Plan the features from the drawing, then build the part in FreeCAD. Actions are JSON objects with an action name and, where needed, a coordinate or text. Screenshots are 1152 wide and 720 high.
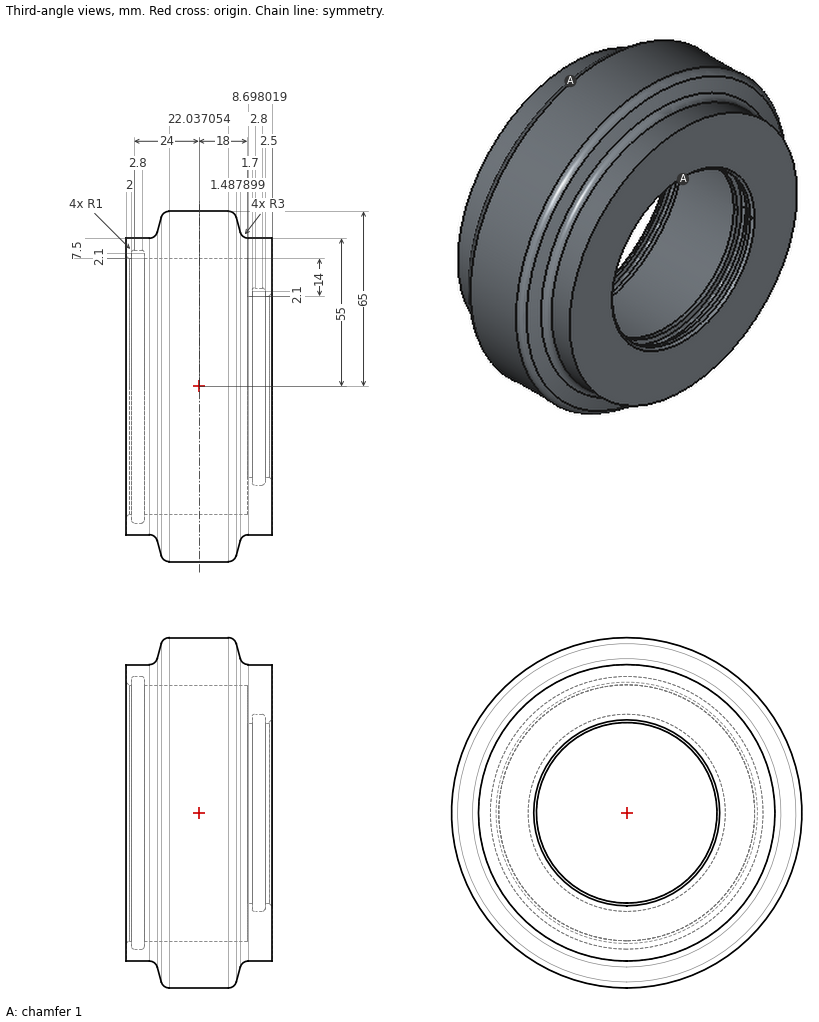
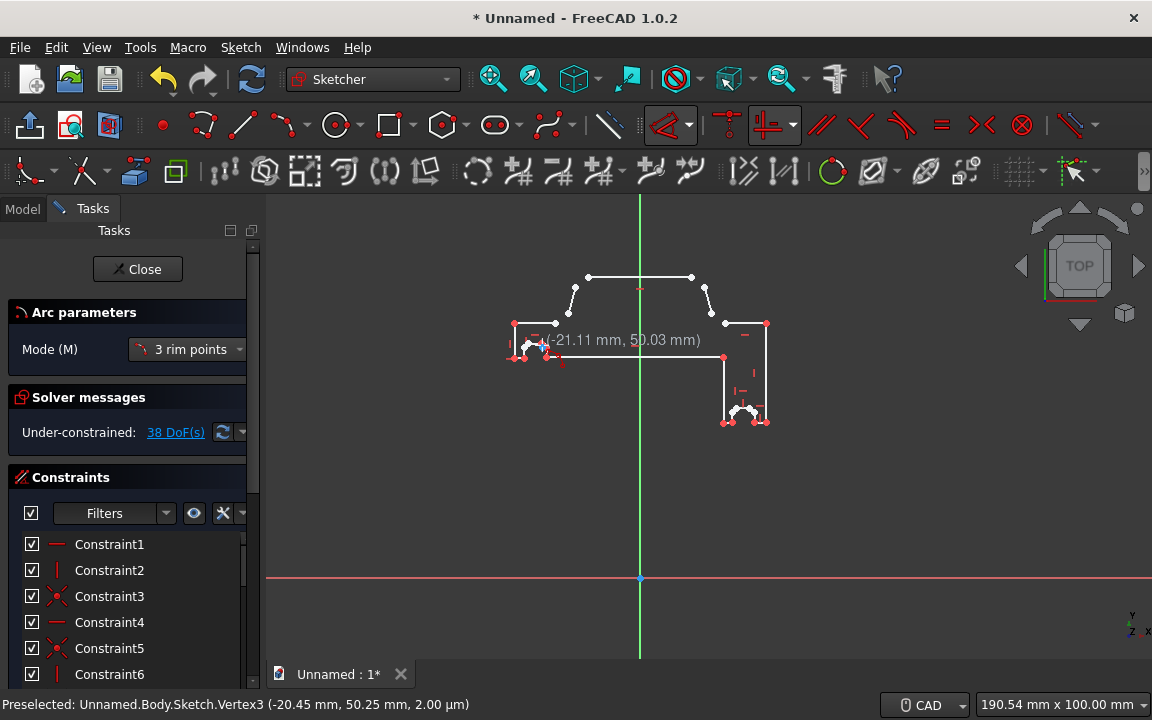
{"action": "scroll", "coordinate": [732, 412], "scroll_direction": "up", "scroll_amount": 6}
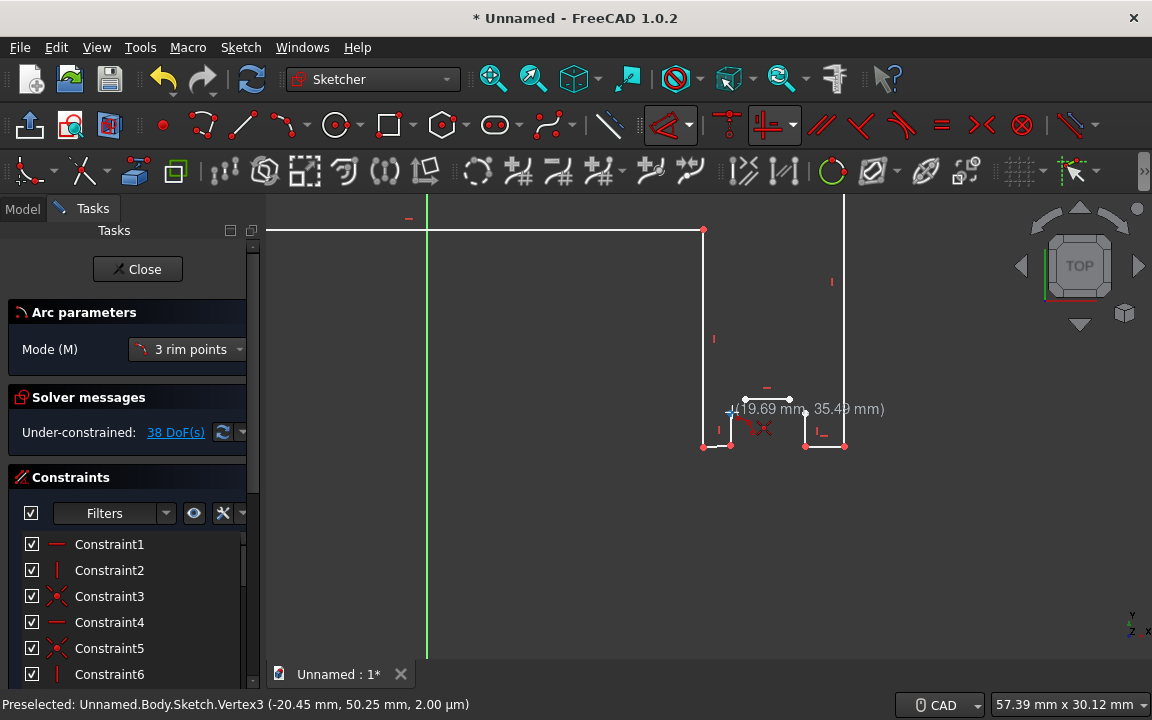
{"action": "left_click", "coordinate": [731, 414]}
{"action": "left_click", "coordinate": [746, 399]}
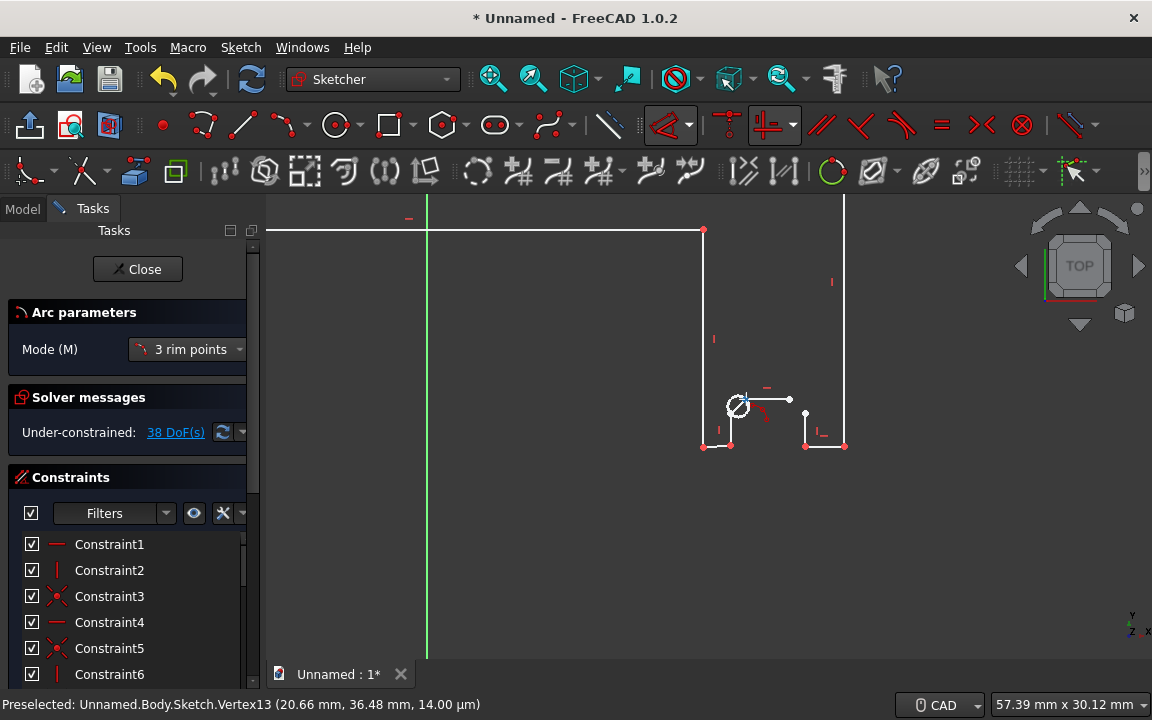
{"action": "scroll", "coordinate": [735, 402], "scroll_direction": "up", "scroll_amount": 7}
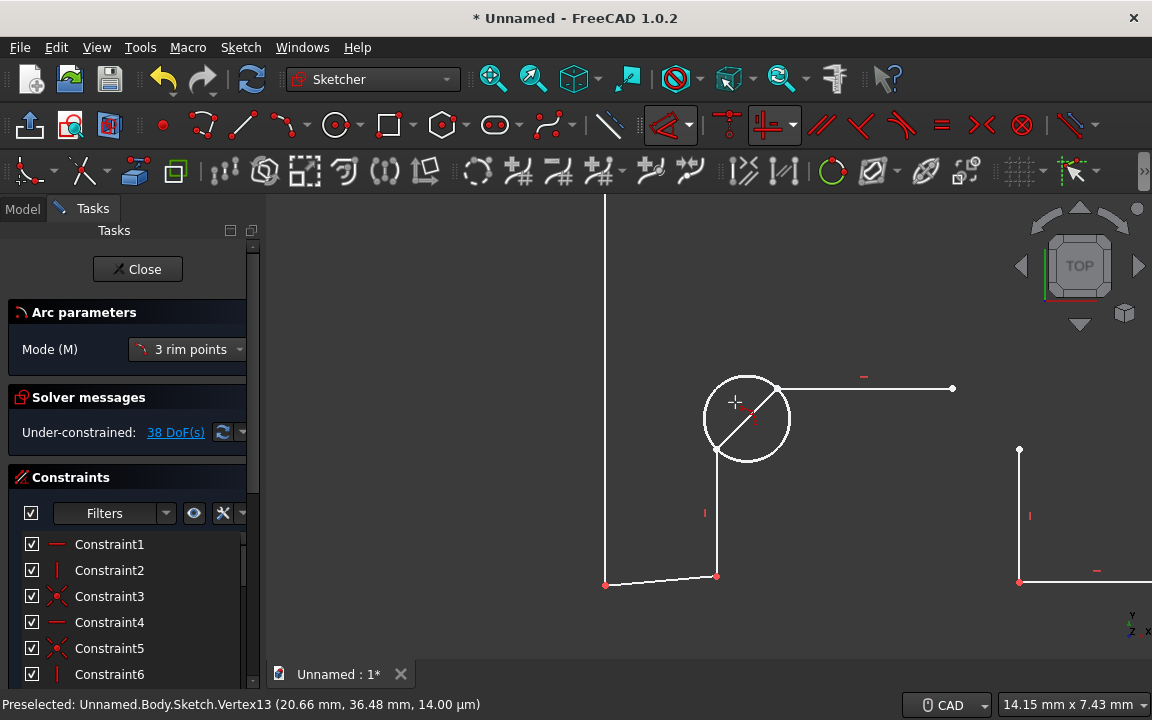
{"action": "left_click", "coordinate": [735, 399]}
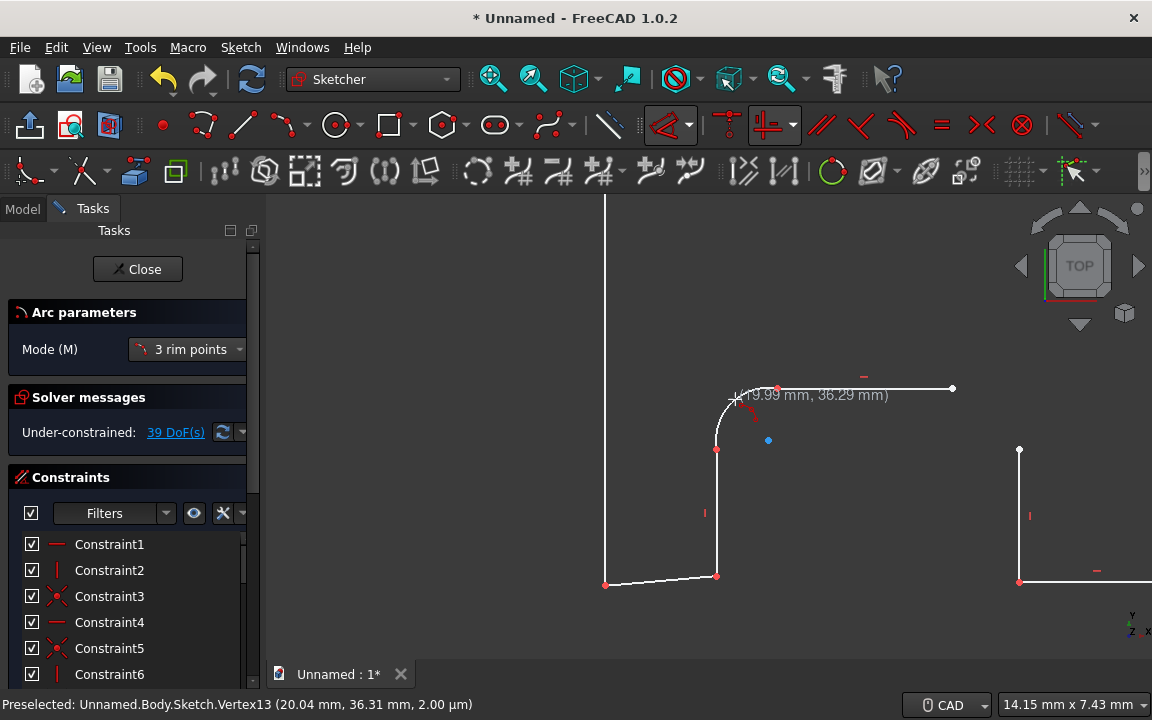
{"action": "scroll", "coordinate": [733, 410], "scroll_direction": "down", "scroll_amount": 13}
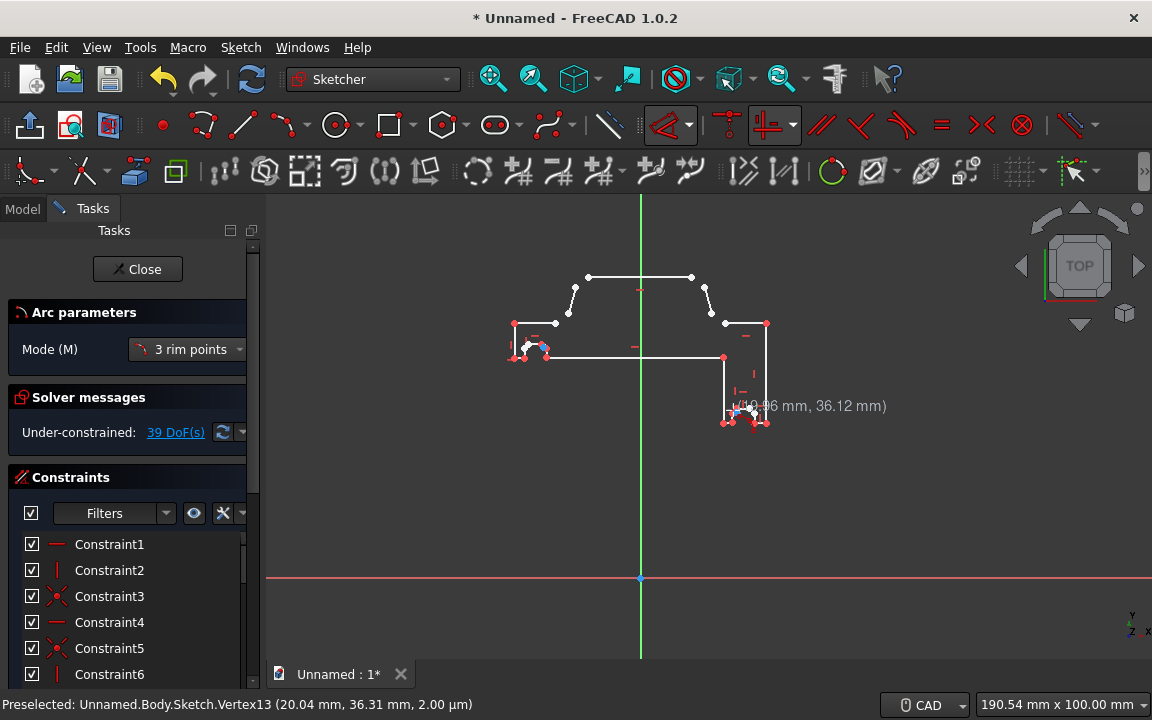
{"action": "scroll", "coordinate": [750, 408], "scroll_direction": "up", "scroll_amount": 5}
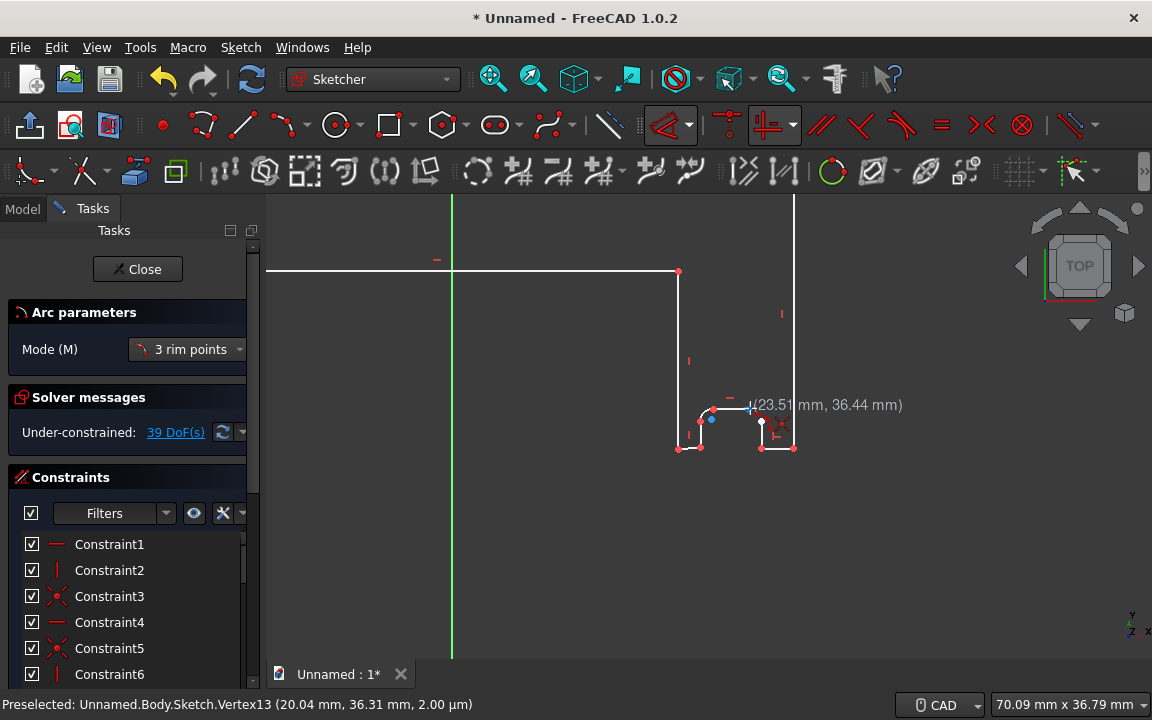
{"action": "left_click", "coordinate": [749, 409]}
{"action": "left_click", "coordinate": [762, 422]}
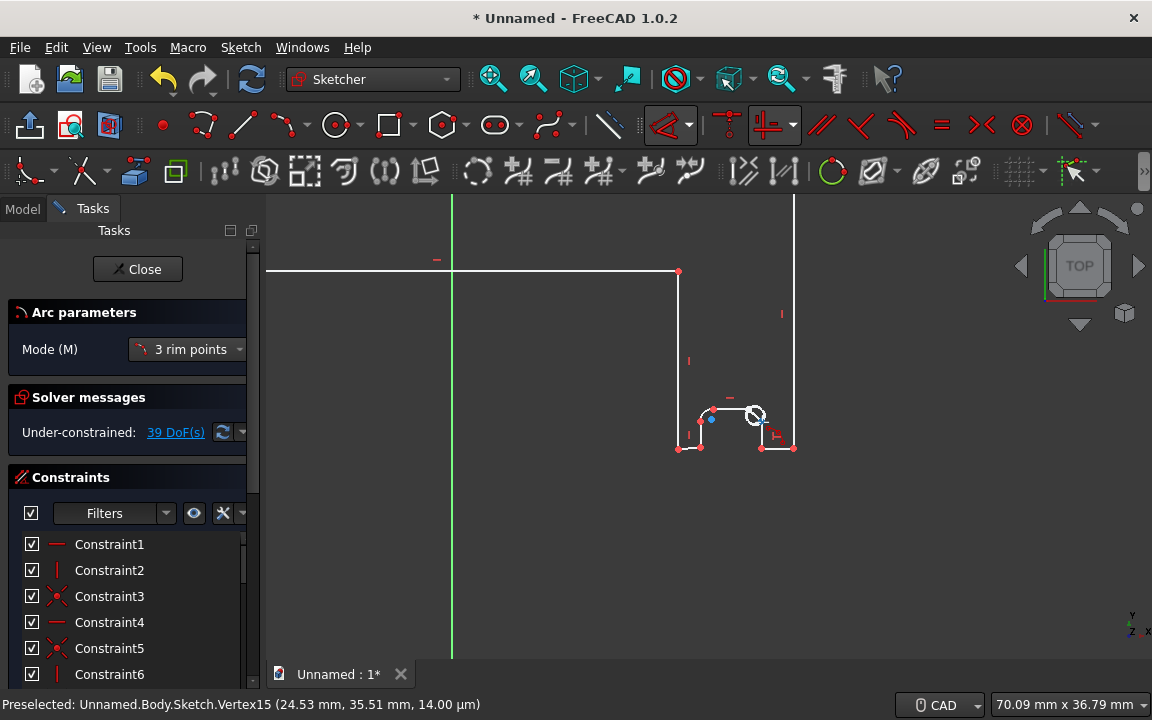
{"action": "scroll", "coordinate": [758, 412], "scroll_direction": "up", "scroll_amount": 8}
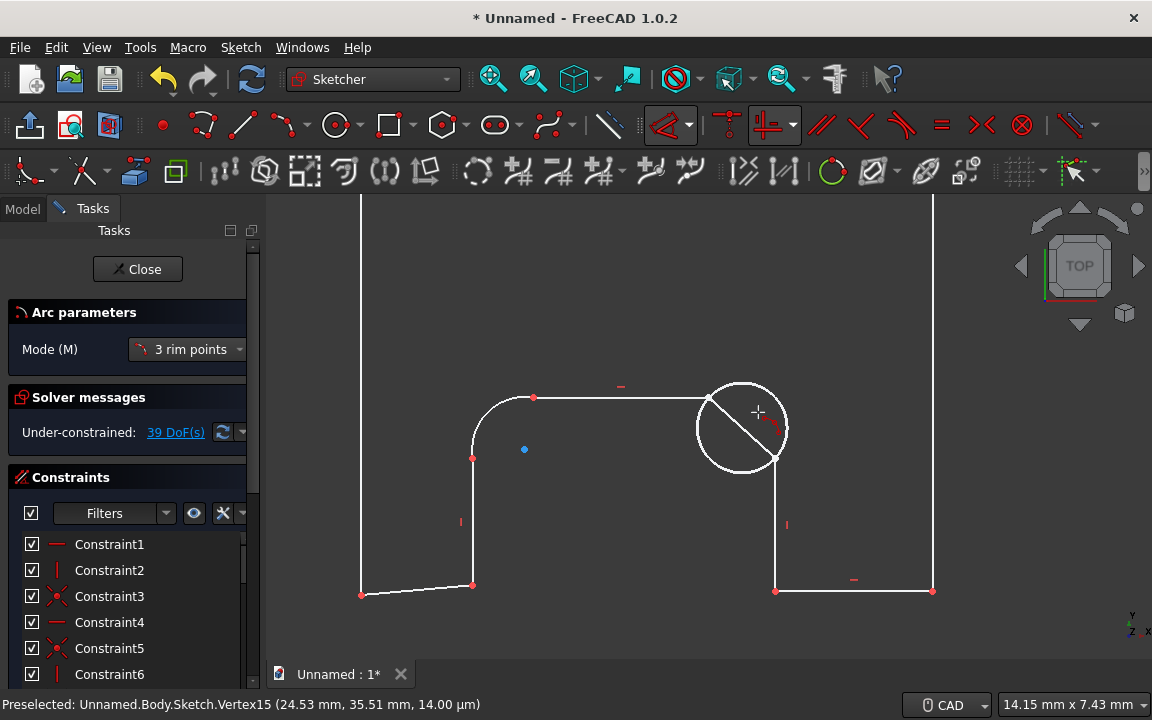
{"action": "left_click", "coordinate": [755, 408]}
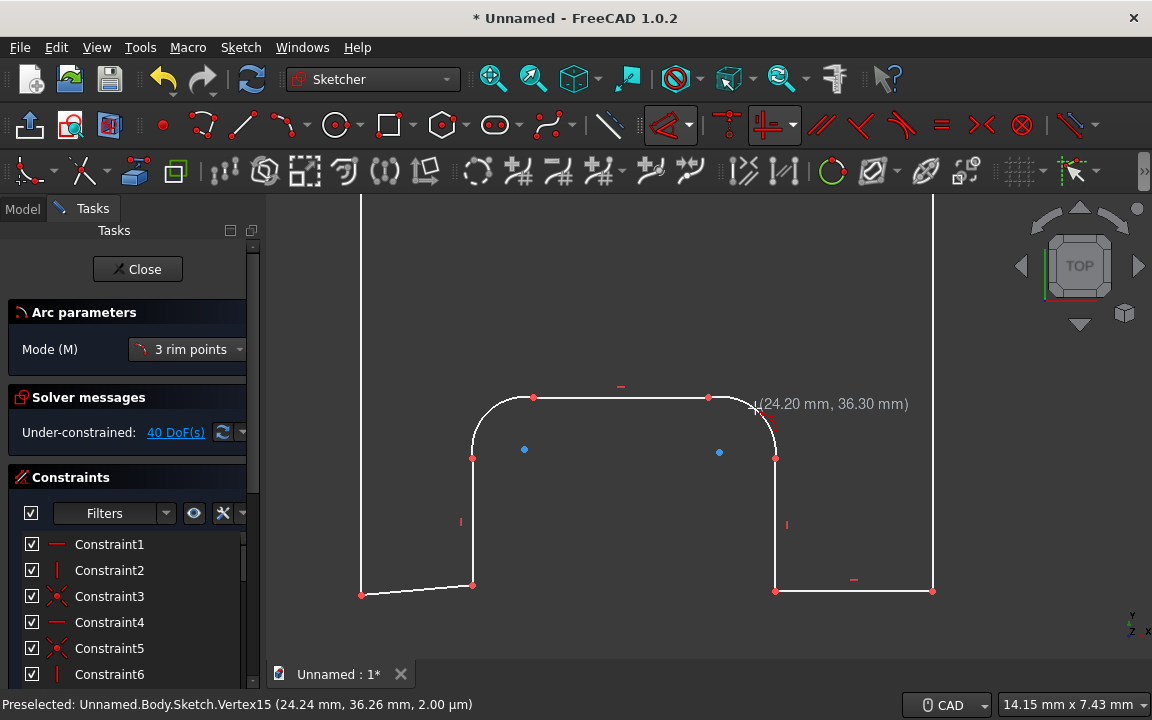
{"action": "scroll", "coordinate": [753, 409], "scroll_direction": "down", "scroll_amount": 13}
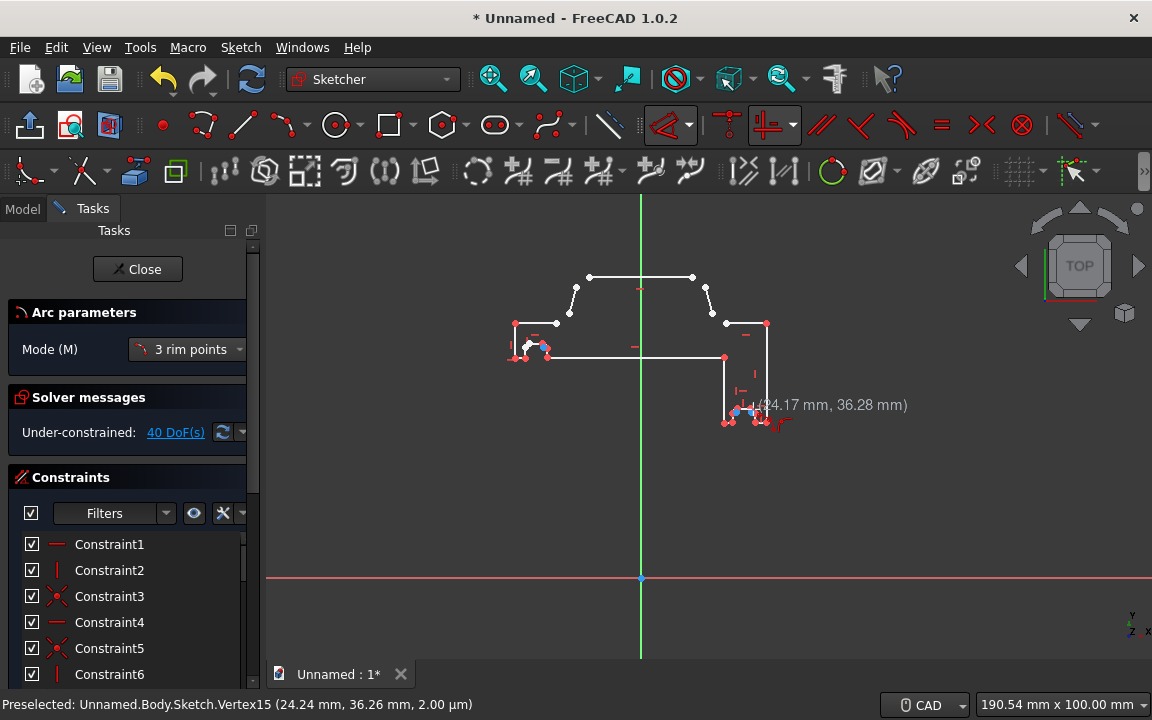
{"action": "left_click", "coordinate": [726, 323]}
{"action": "left_click", "coordinate": [712, 313]}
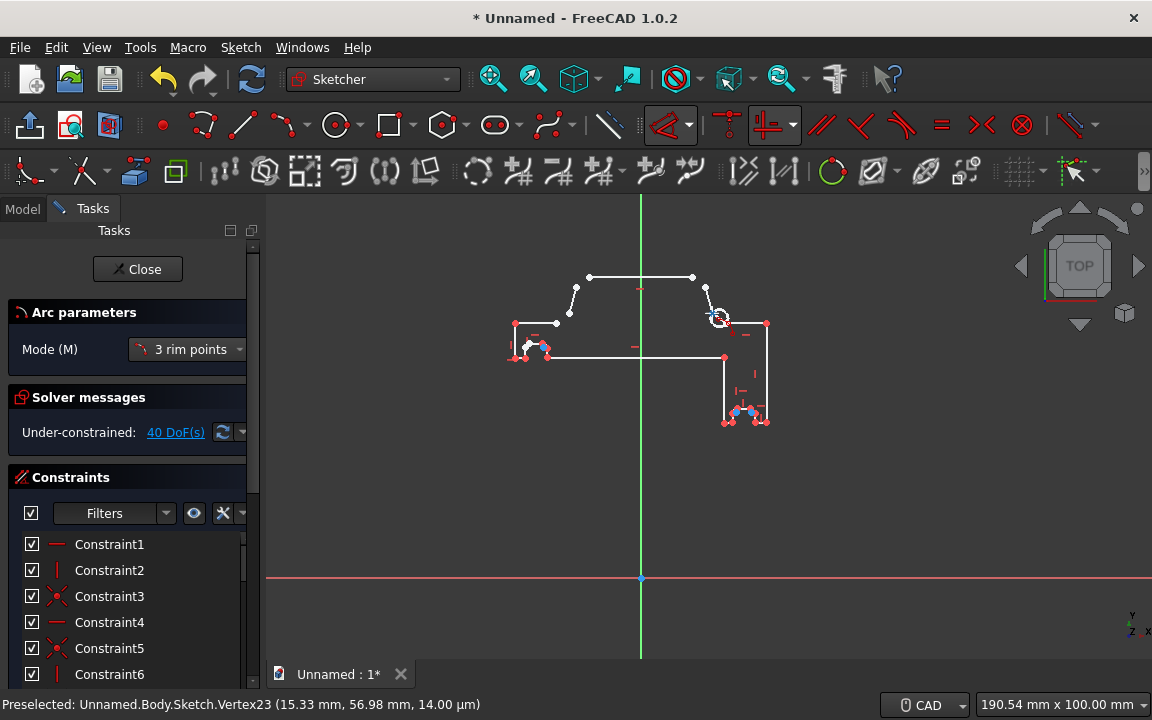
{"action": "scroll", "coordinate": [718, 320], "scroll_direction": "up", "scroll_amount": 9}